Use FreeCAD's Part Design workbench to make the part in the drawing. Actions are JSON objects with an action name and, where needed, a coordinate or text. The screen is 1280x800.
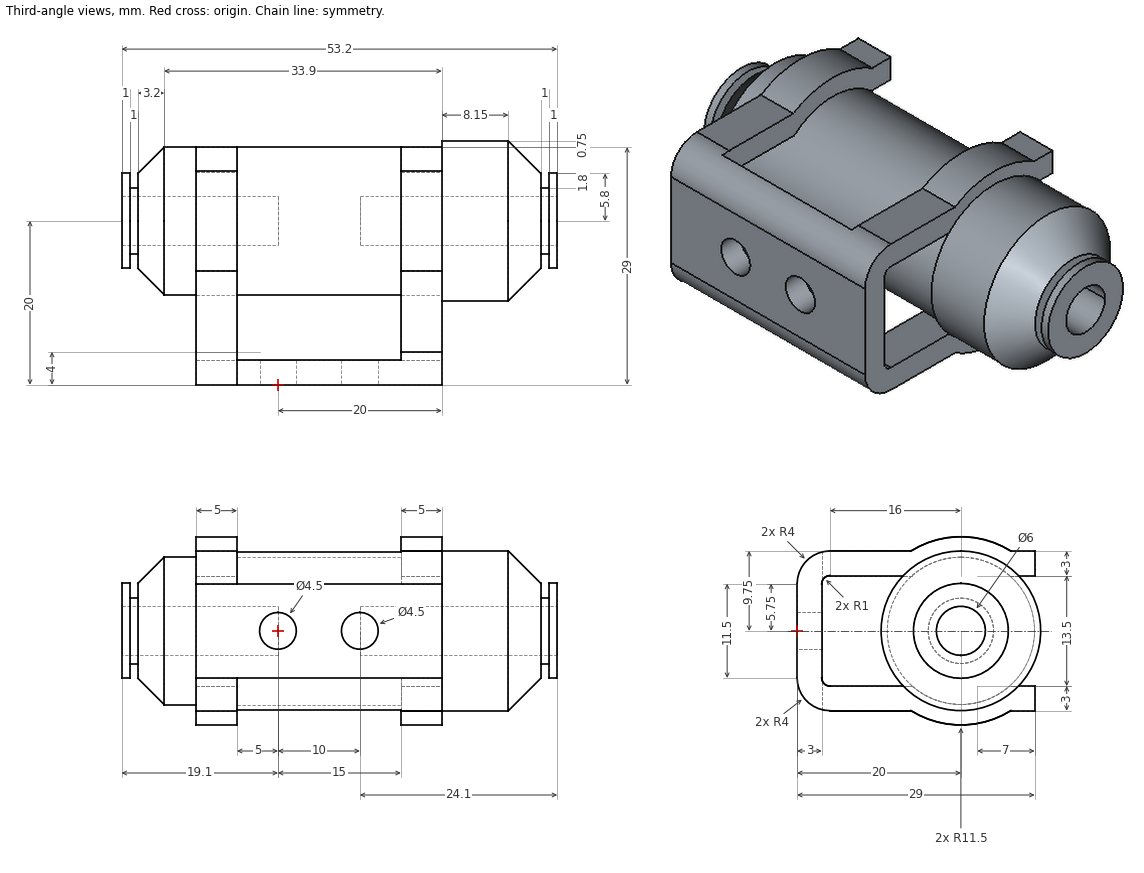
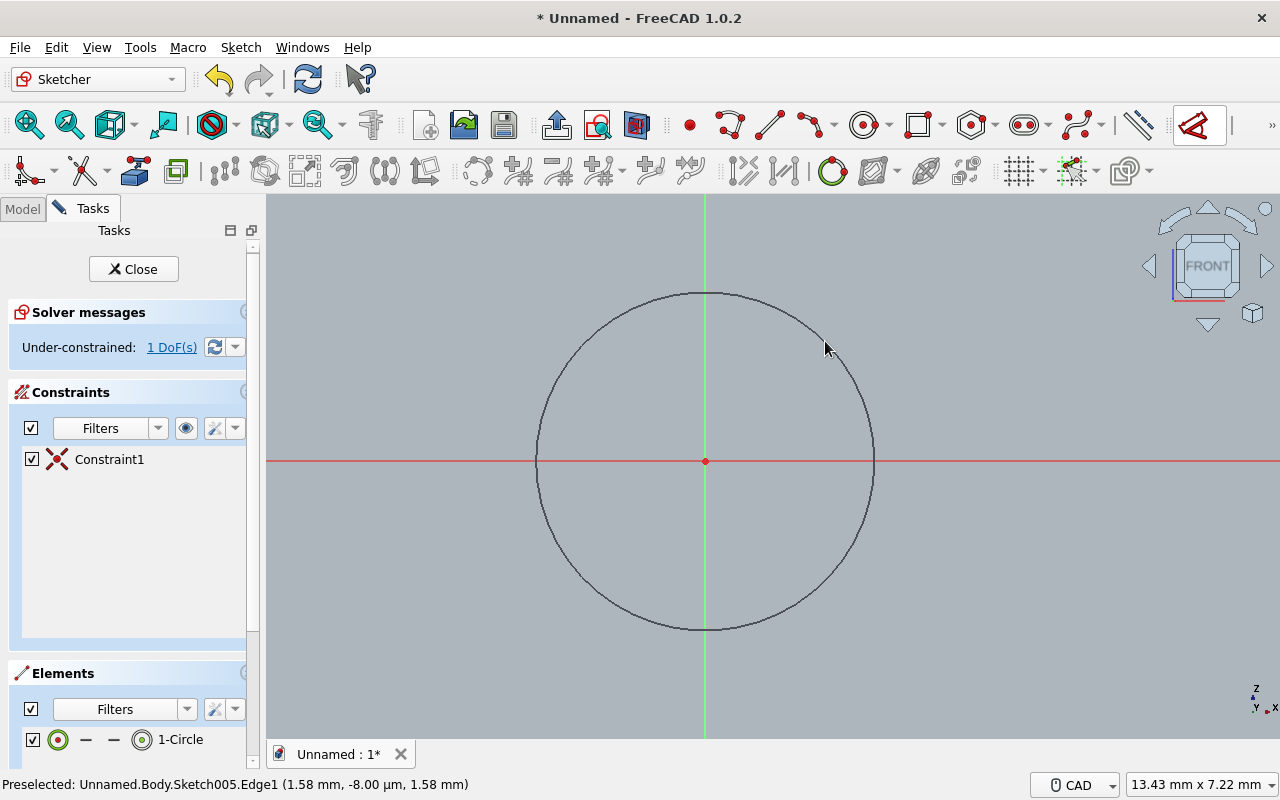
{"action": "left_click", "coordinate": [824, 341]}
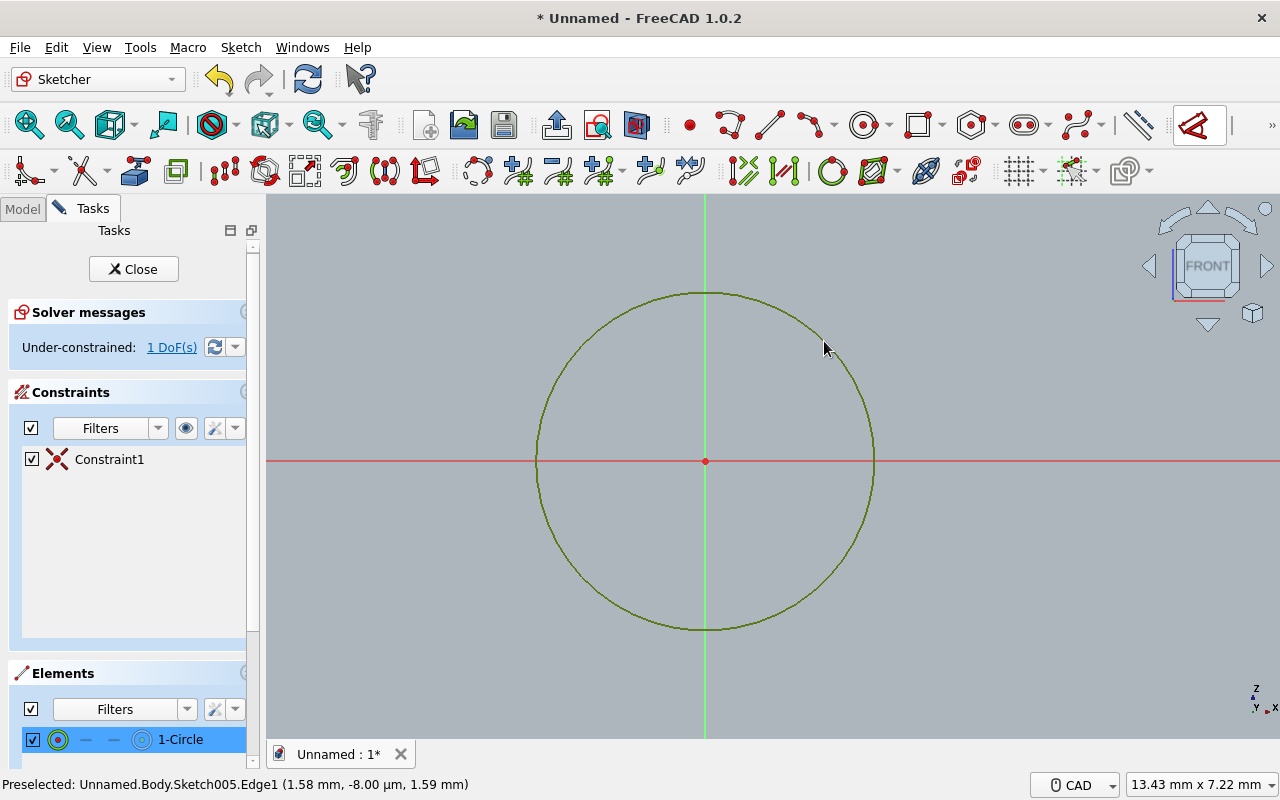
{"action": "left_click", "coordinate": [1220, 126]}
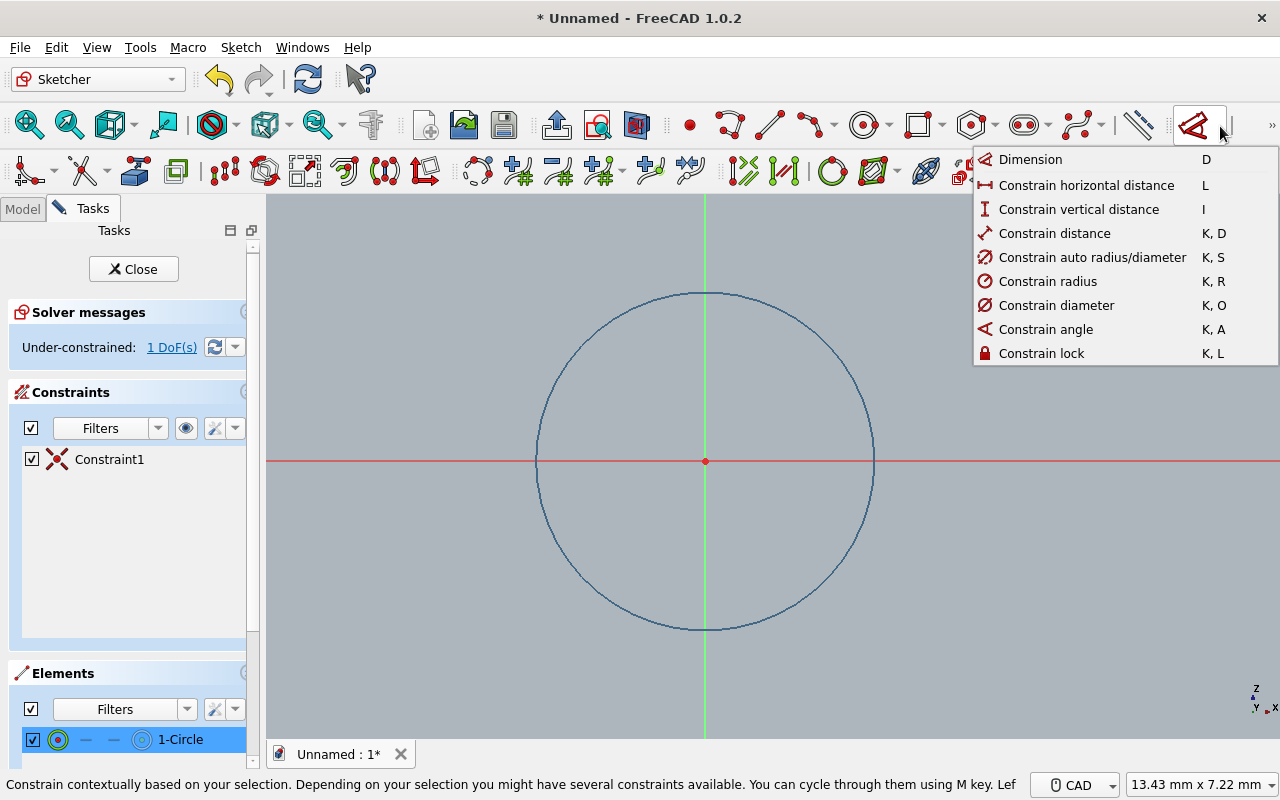
{"action": "left_click", "coordinate": [1126, 305]}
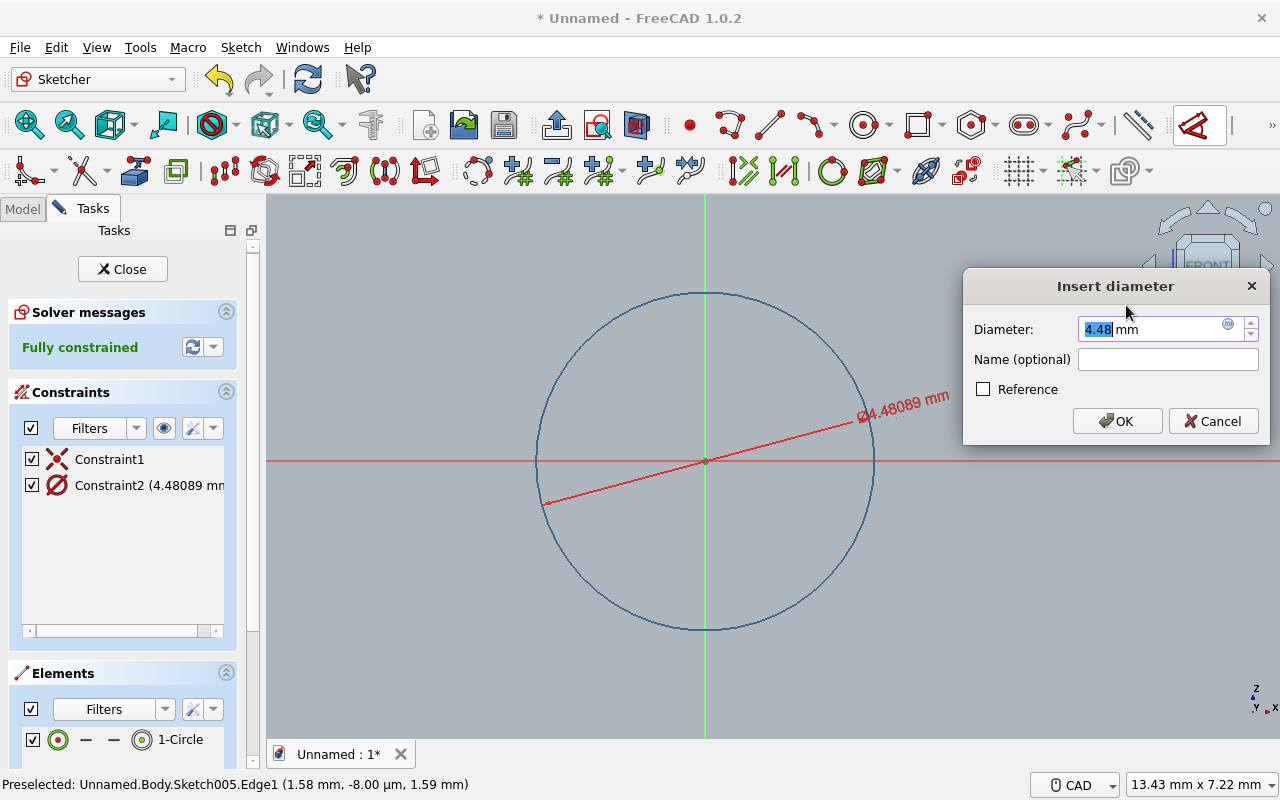
{"action": "type", "text": "4.5"}
{"action": "key", "text": "Return"}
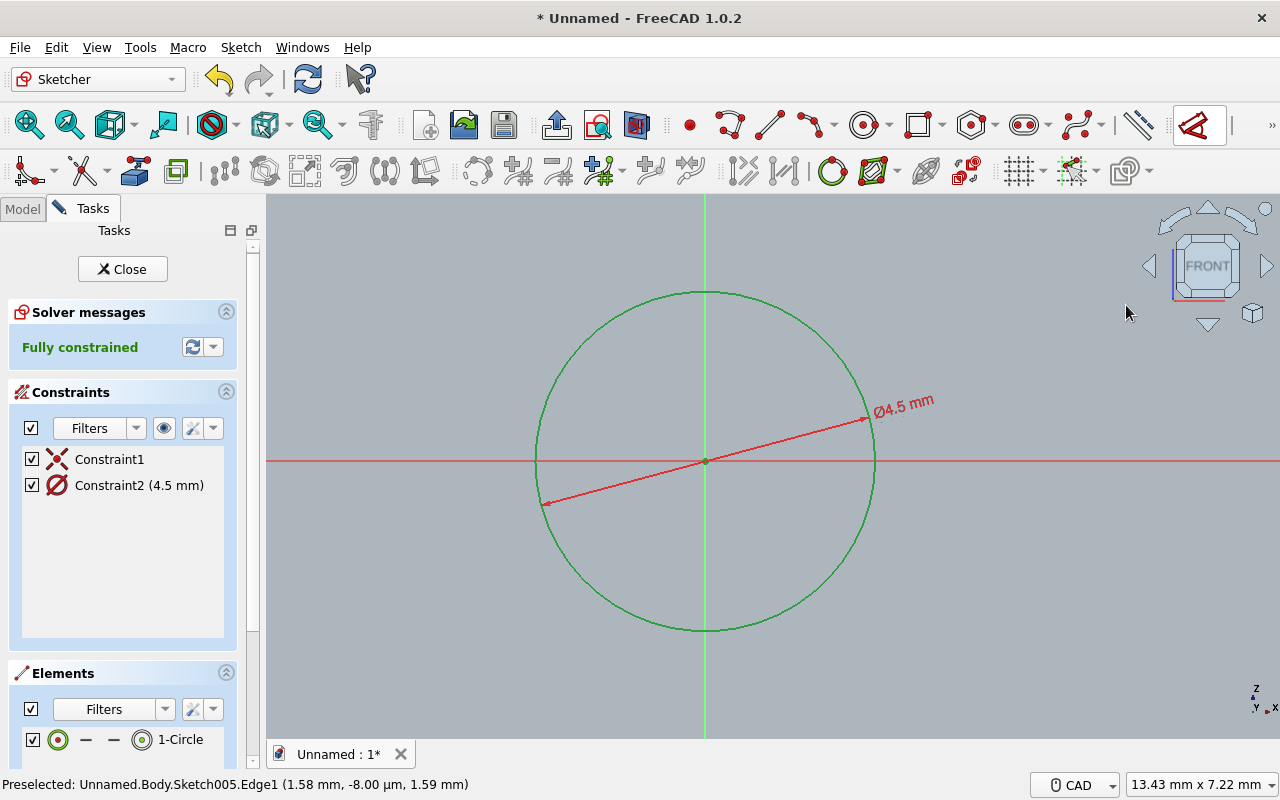
{"action": "left_click", "coordinate": [123, 269]}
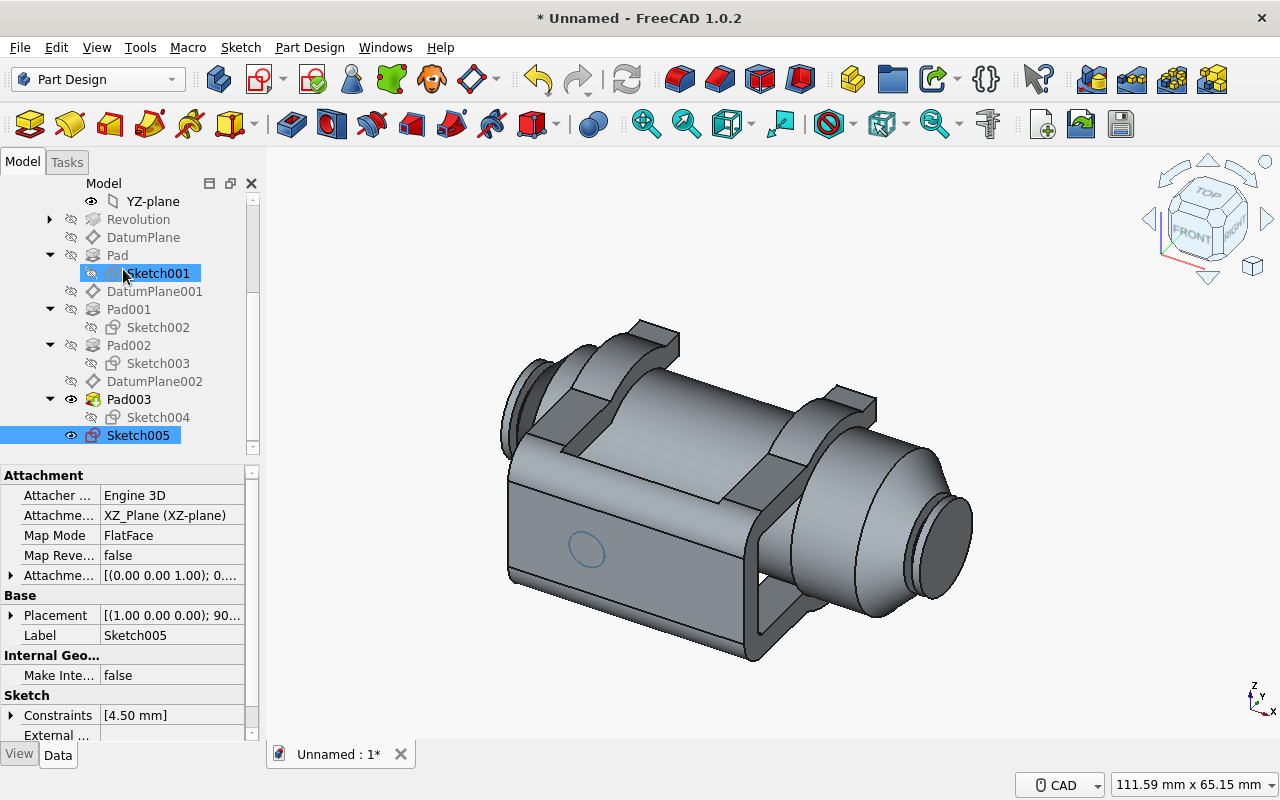
{"action": "left_click", "coordinate": [292, 124]}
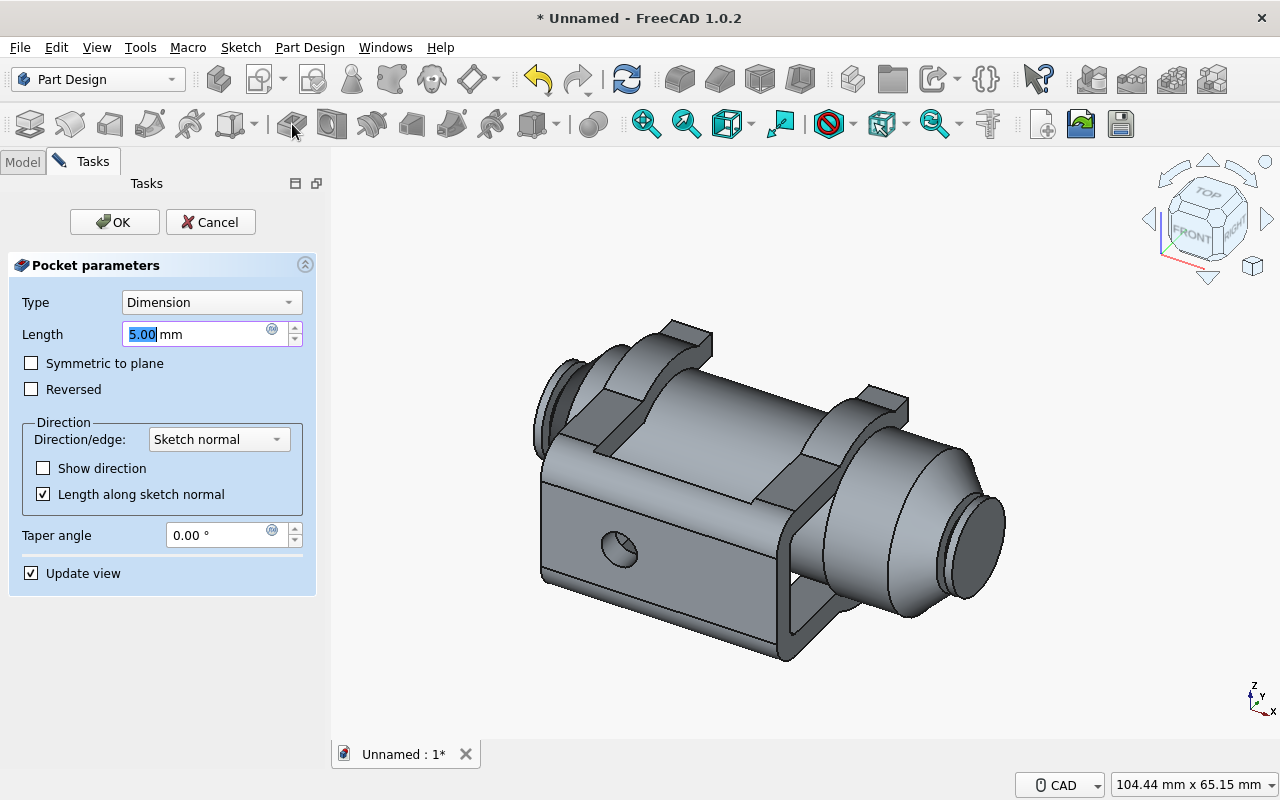
{"action": "type", "text": "4"}
{"action": "key", "text": "Tab"}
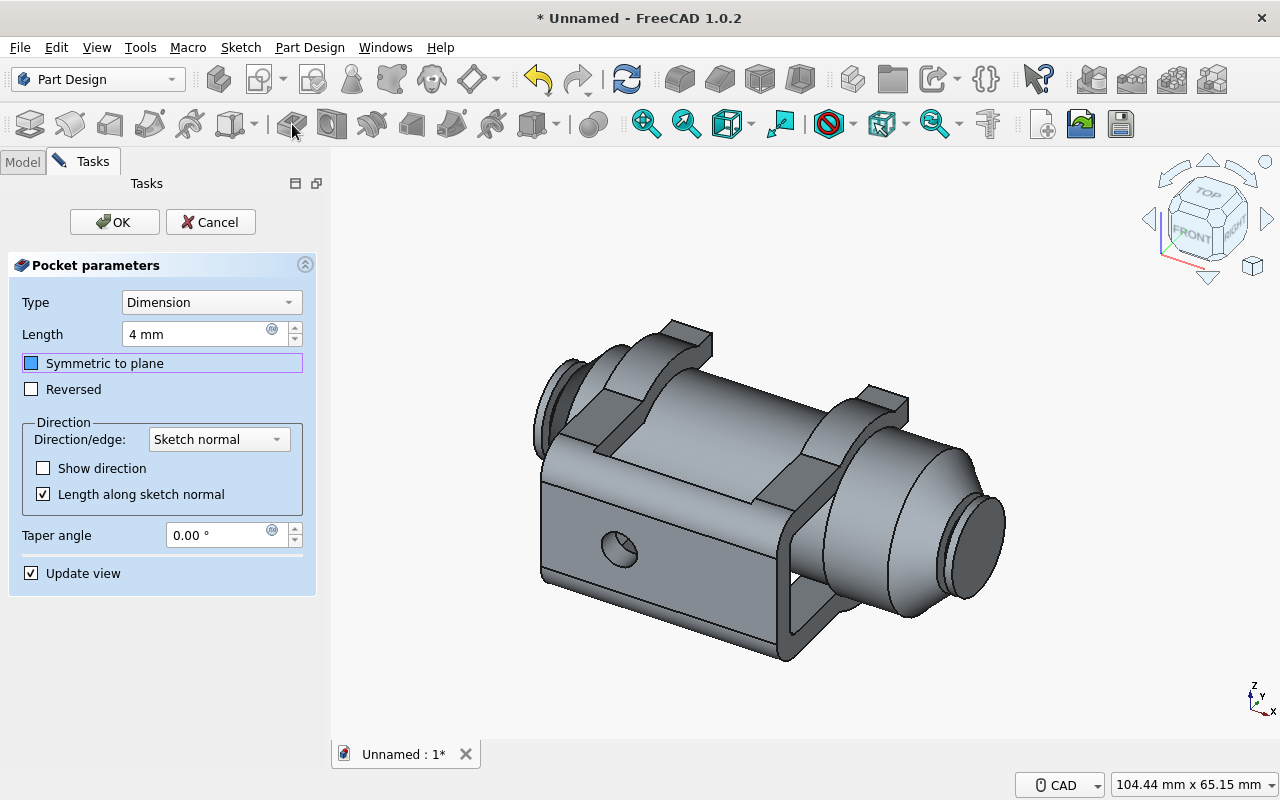
{"action": "left_click", "coordinate": [115, 222]}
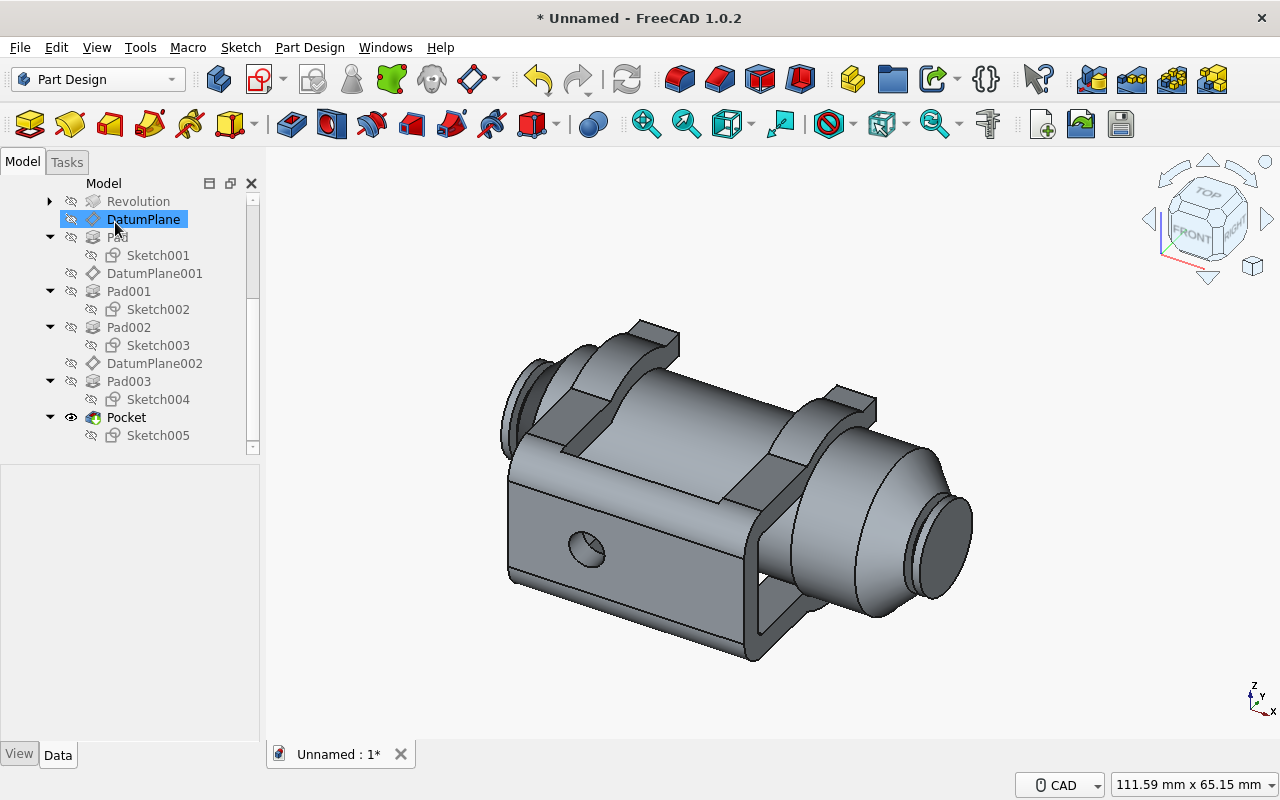
{"action": "left_click", "coordinate": [260, 80]}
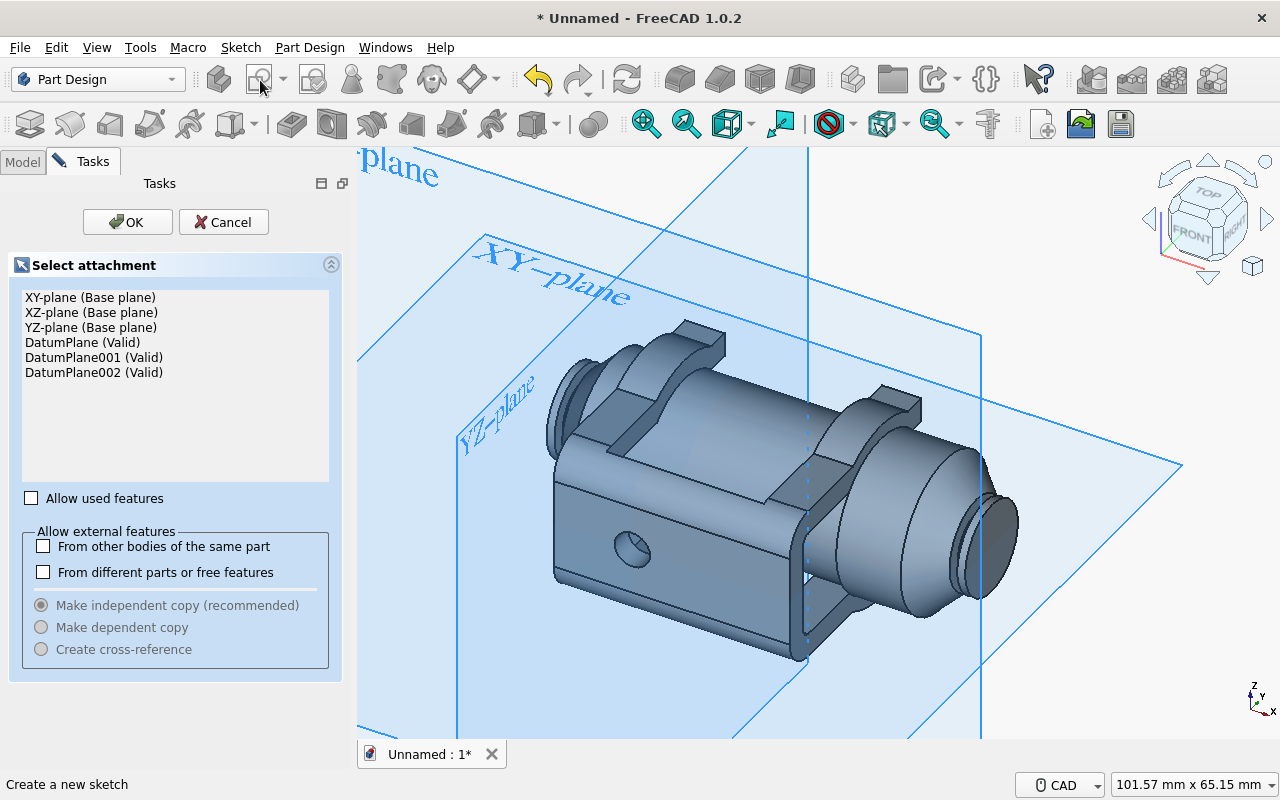
{"action": "left_click", "coordinate": [82, 312]}